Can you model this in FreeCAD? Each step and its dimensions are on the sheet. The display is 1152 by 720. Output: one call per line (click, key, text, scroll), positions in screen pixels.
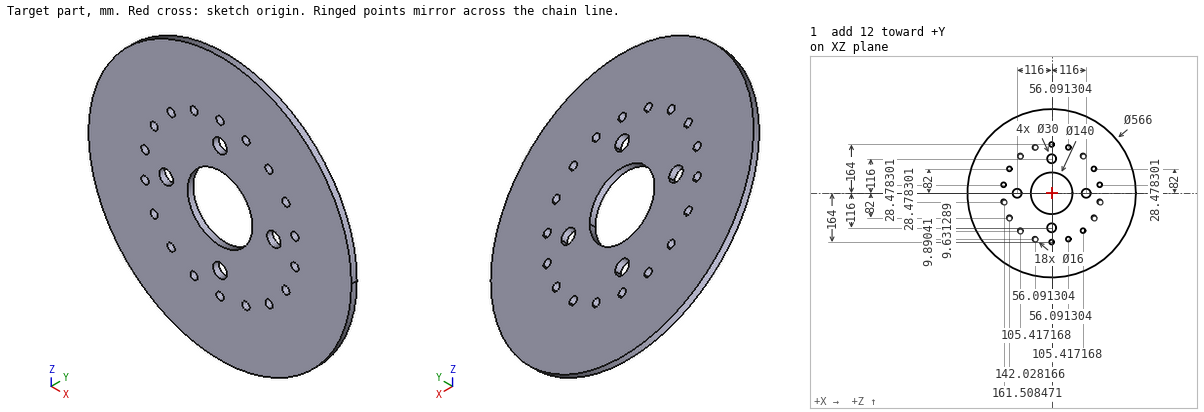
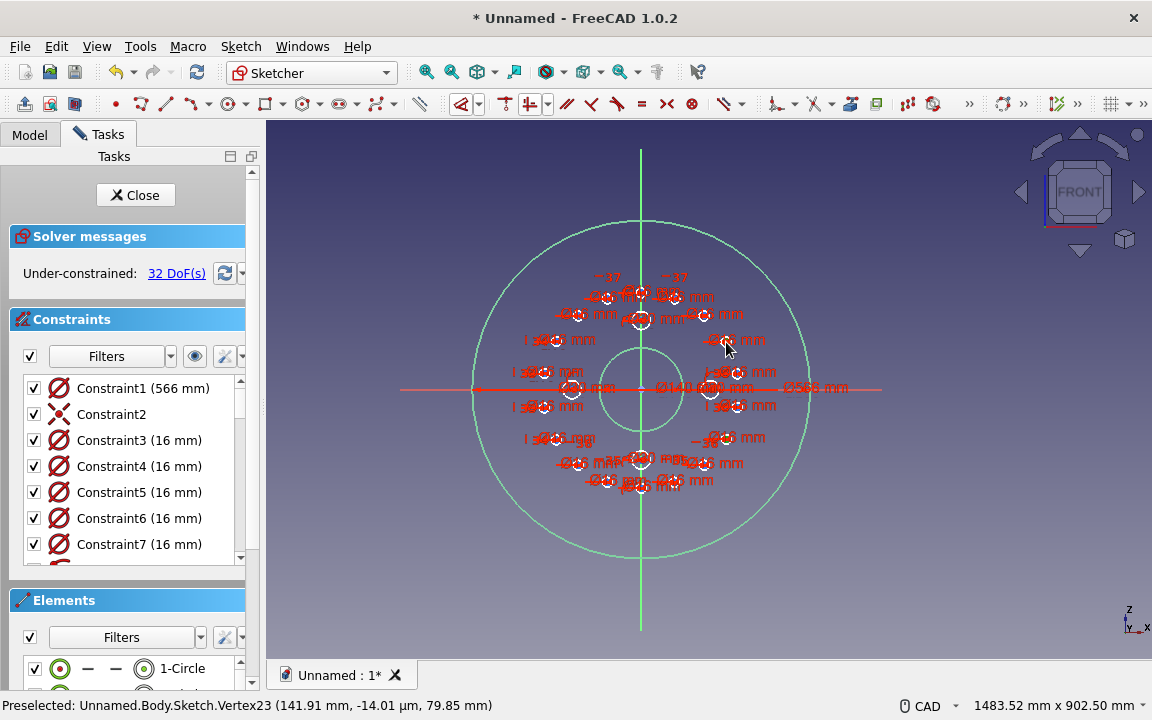
click(548, 104)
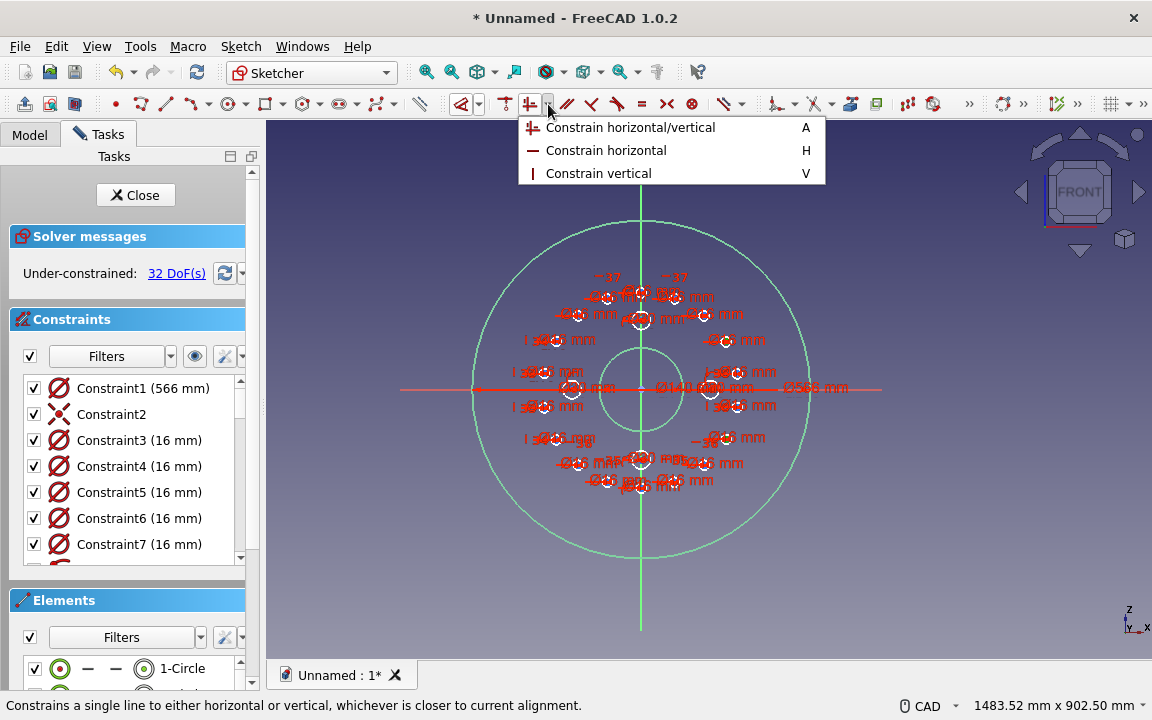
click(672, 174)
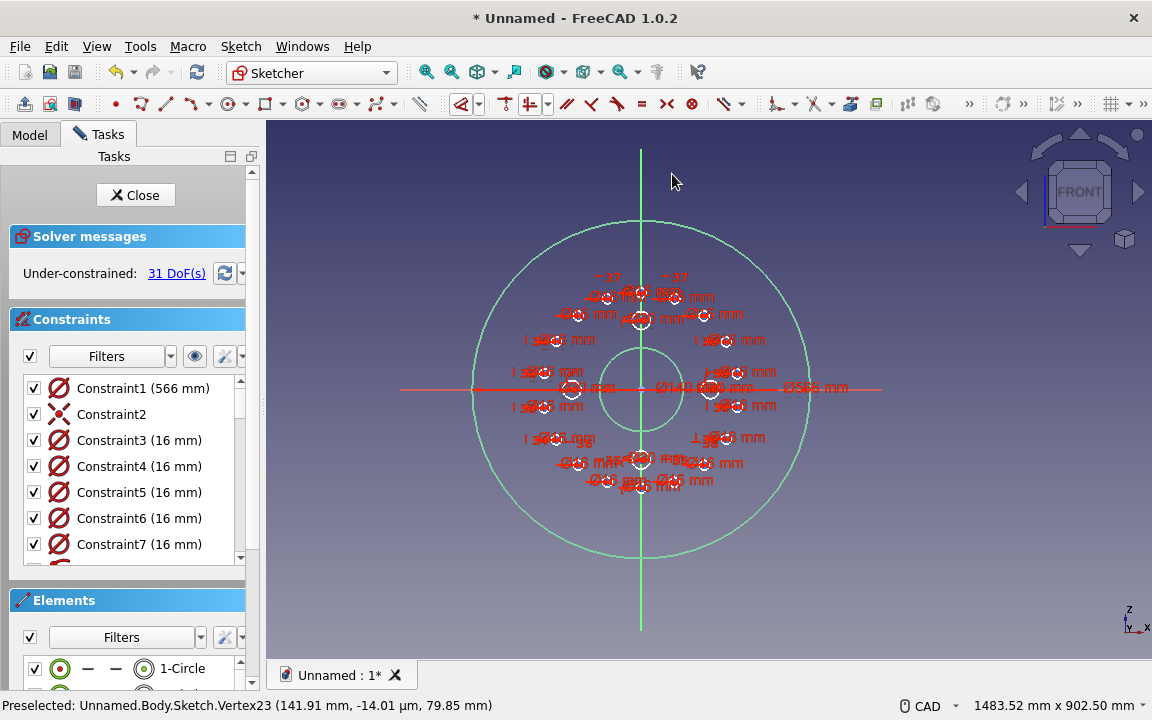
click(578, 465)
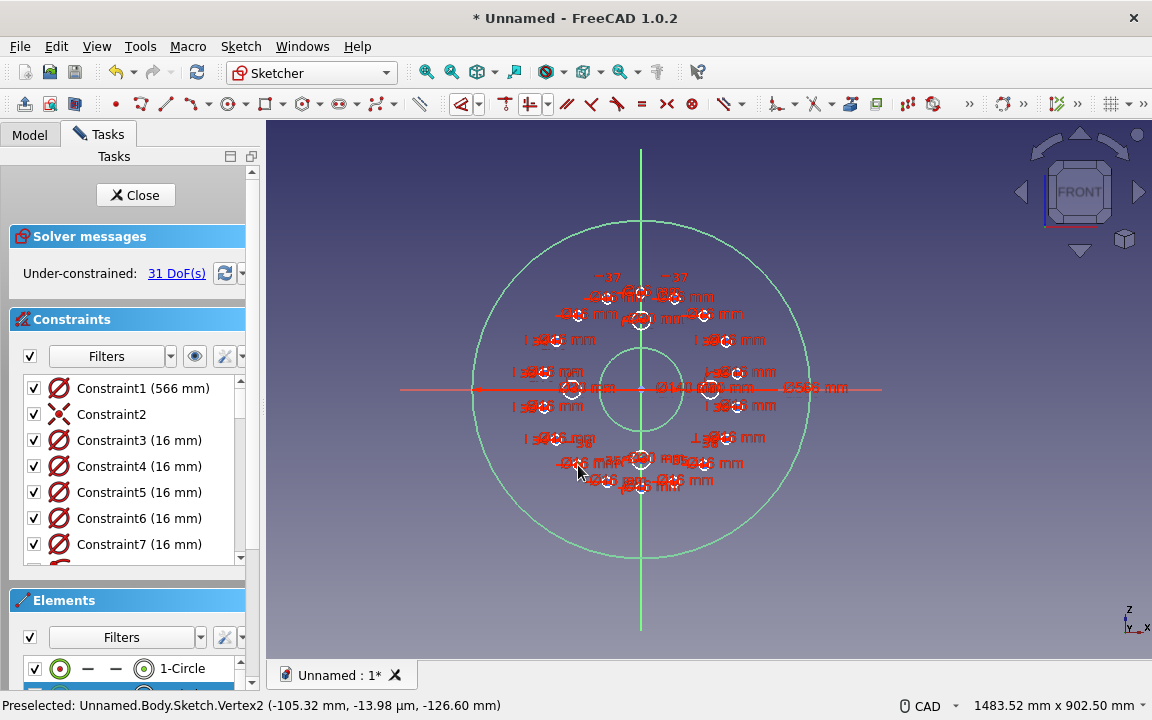
click(578, 316)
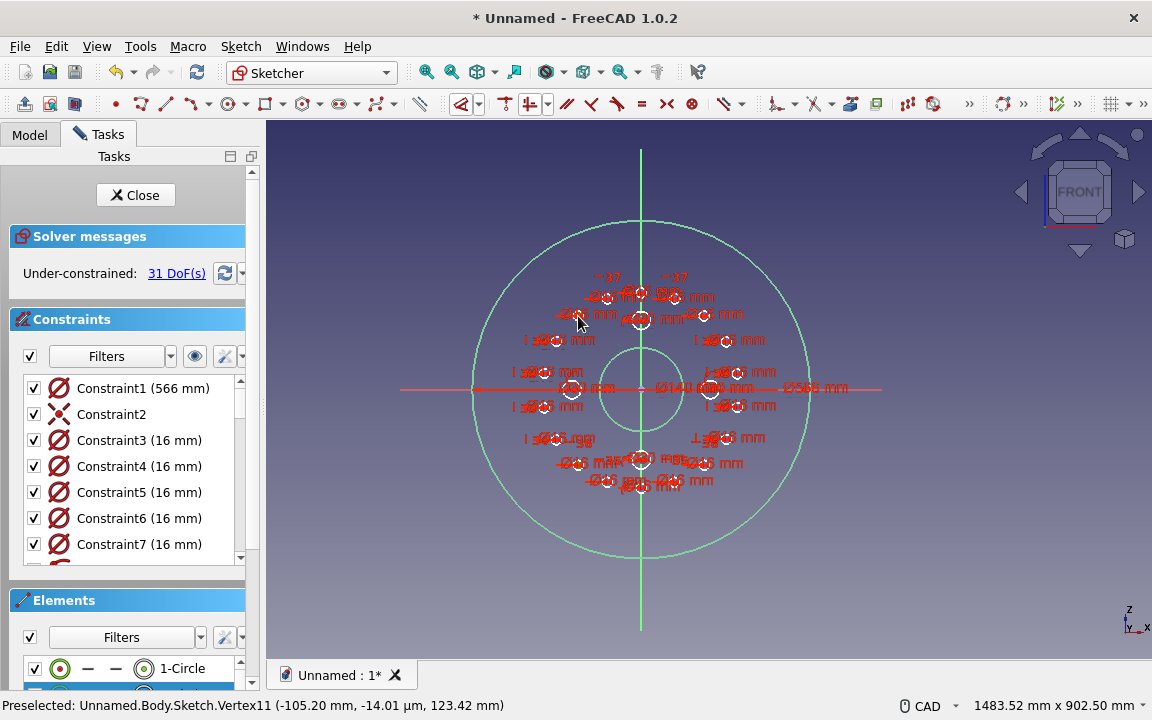
click(442, 390)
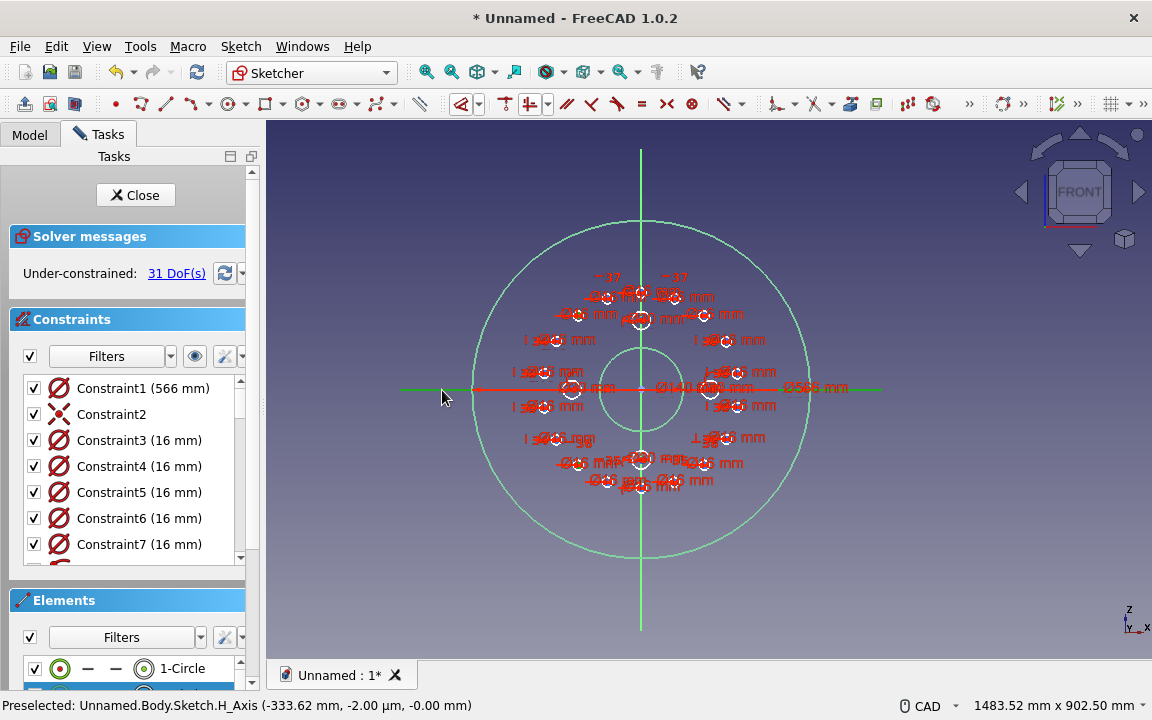
click(667, 104)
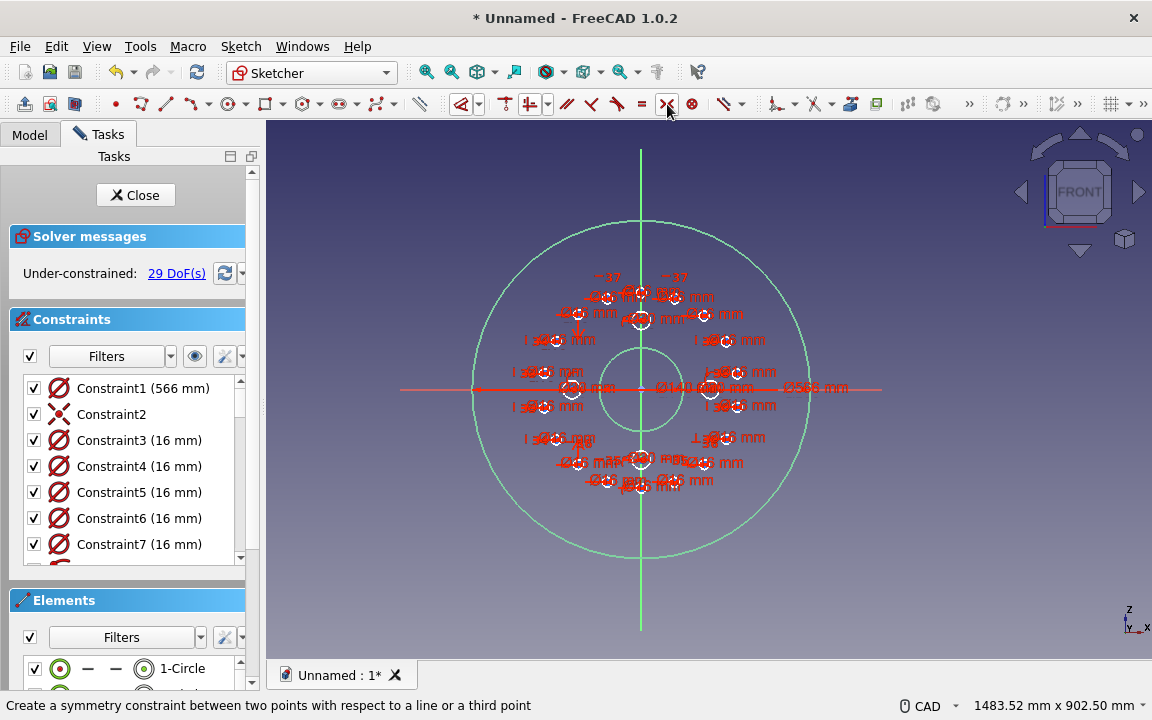
click(607, 482)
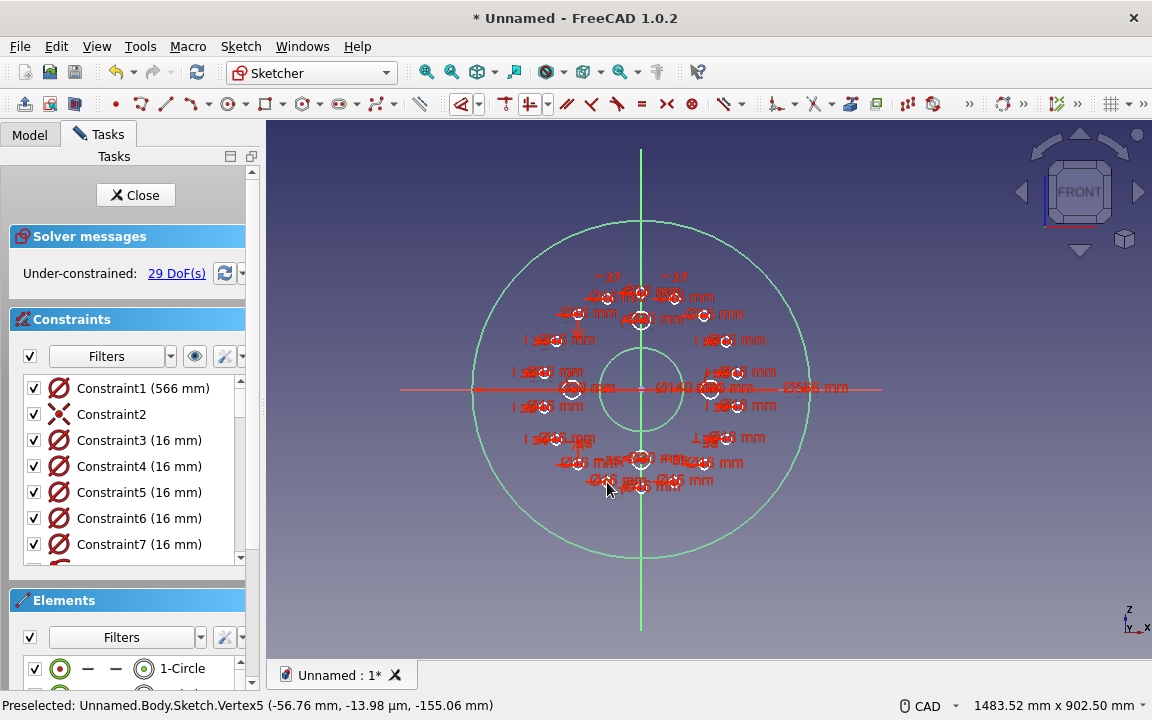
click(607, 299)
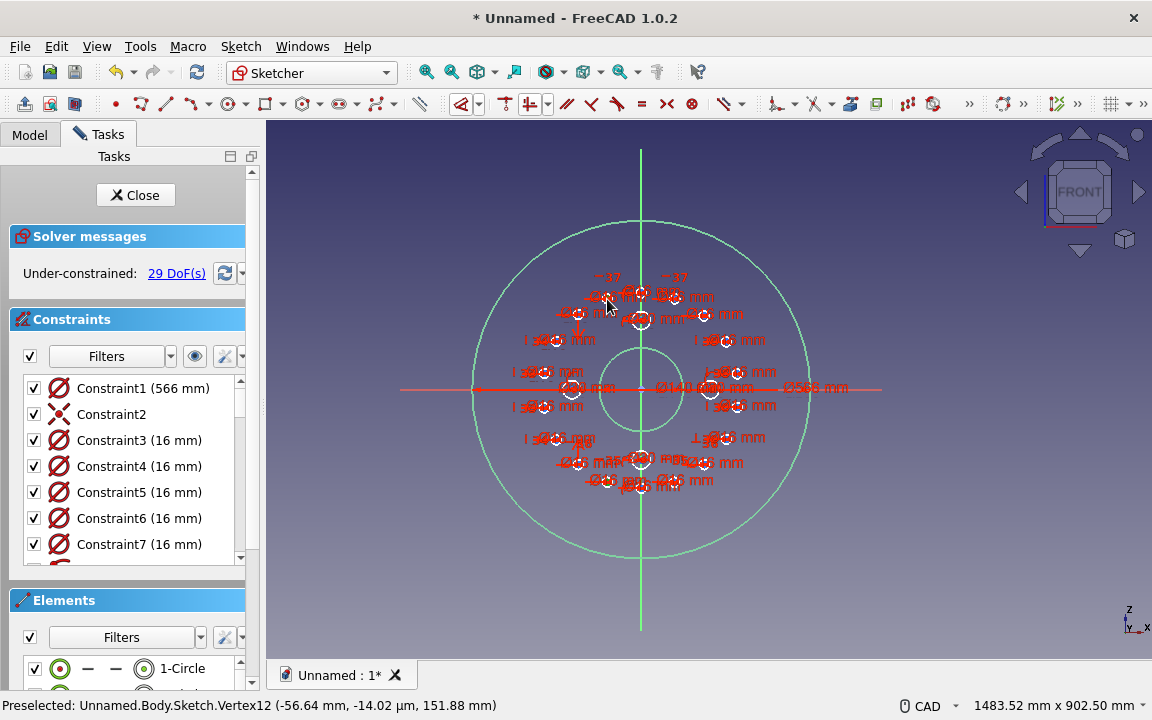
click(442, 390)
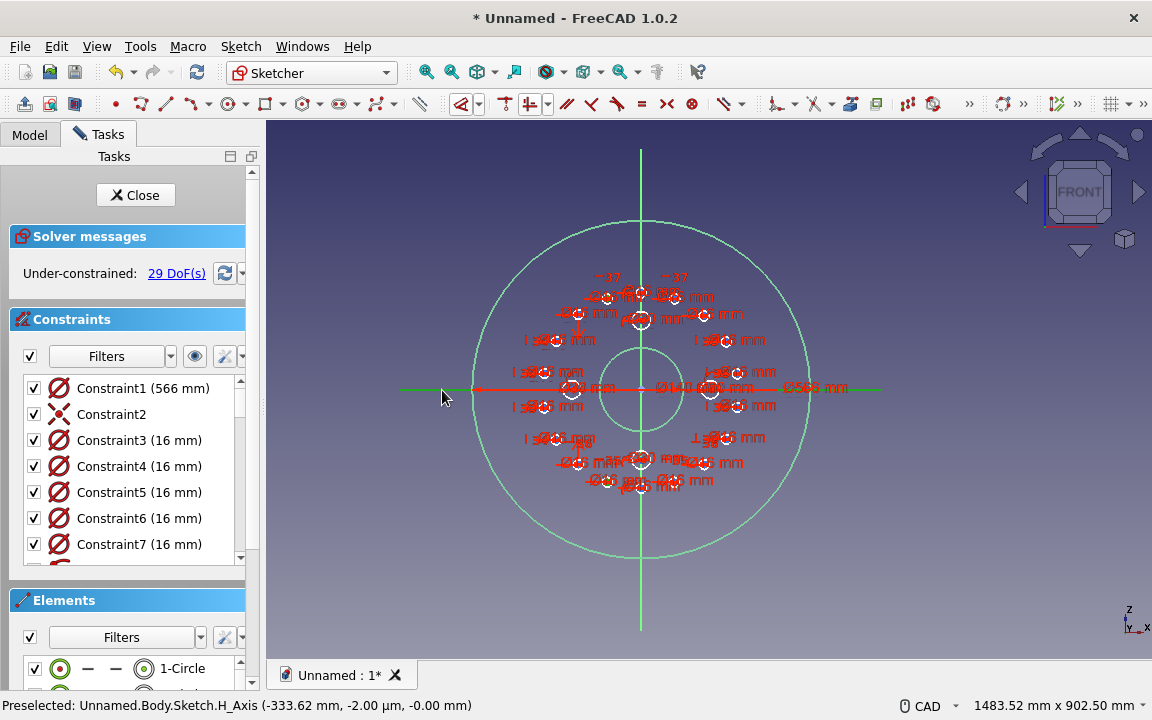
click(667, 104)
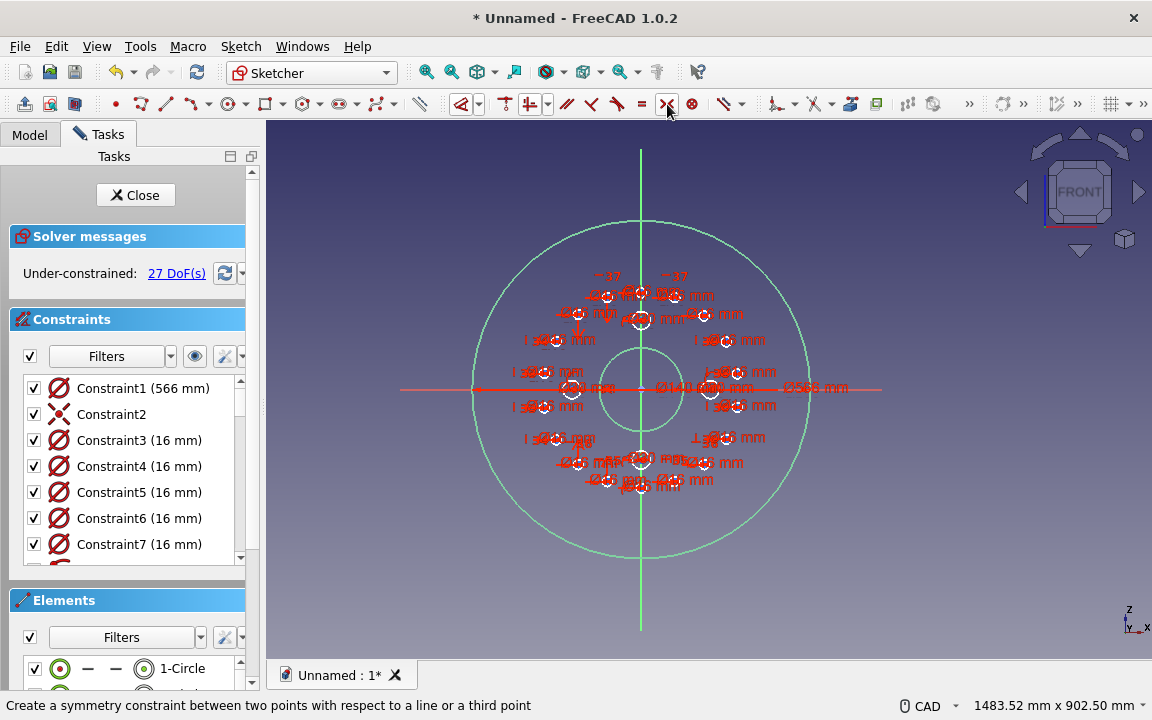
click(556, 440)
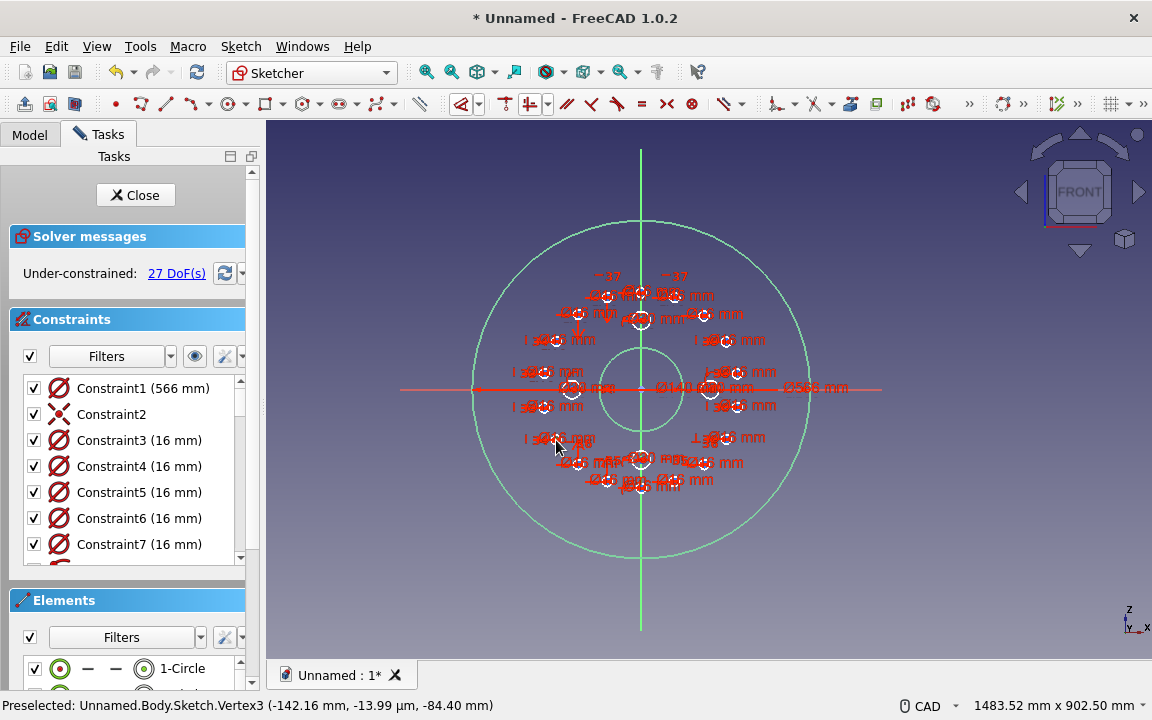
click(726, 439)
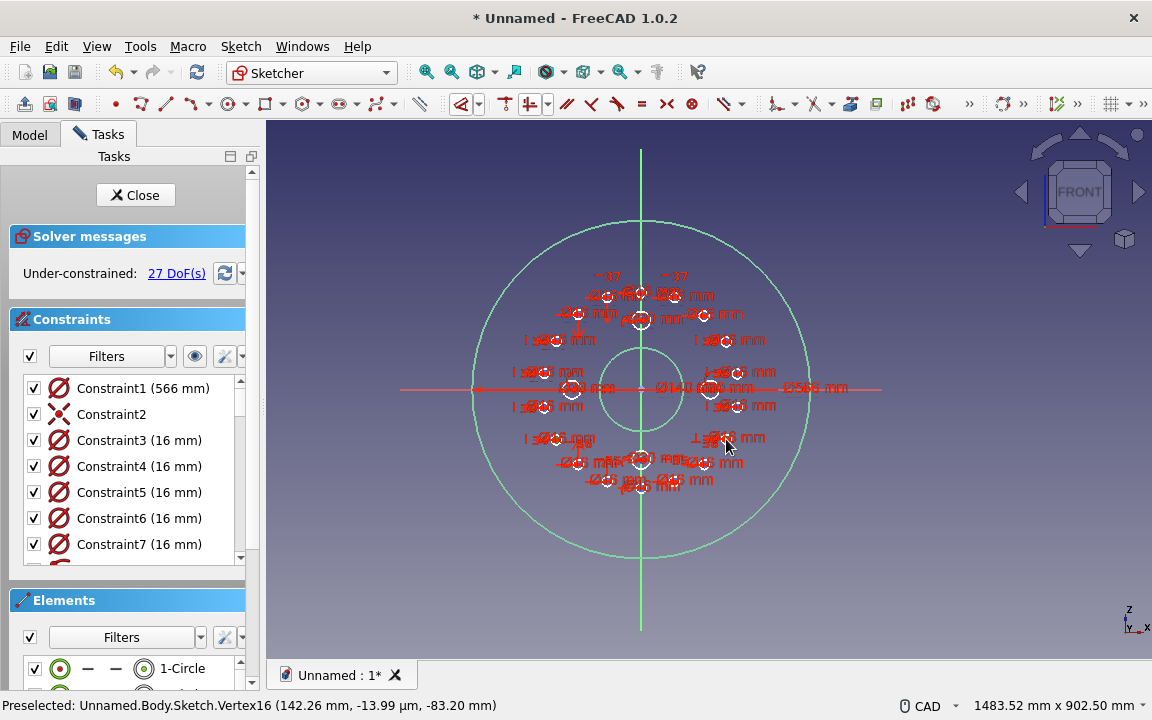
click(641, 596)